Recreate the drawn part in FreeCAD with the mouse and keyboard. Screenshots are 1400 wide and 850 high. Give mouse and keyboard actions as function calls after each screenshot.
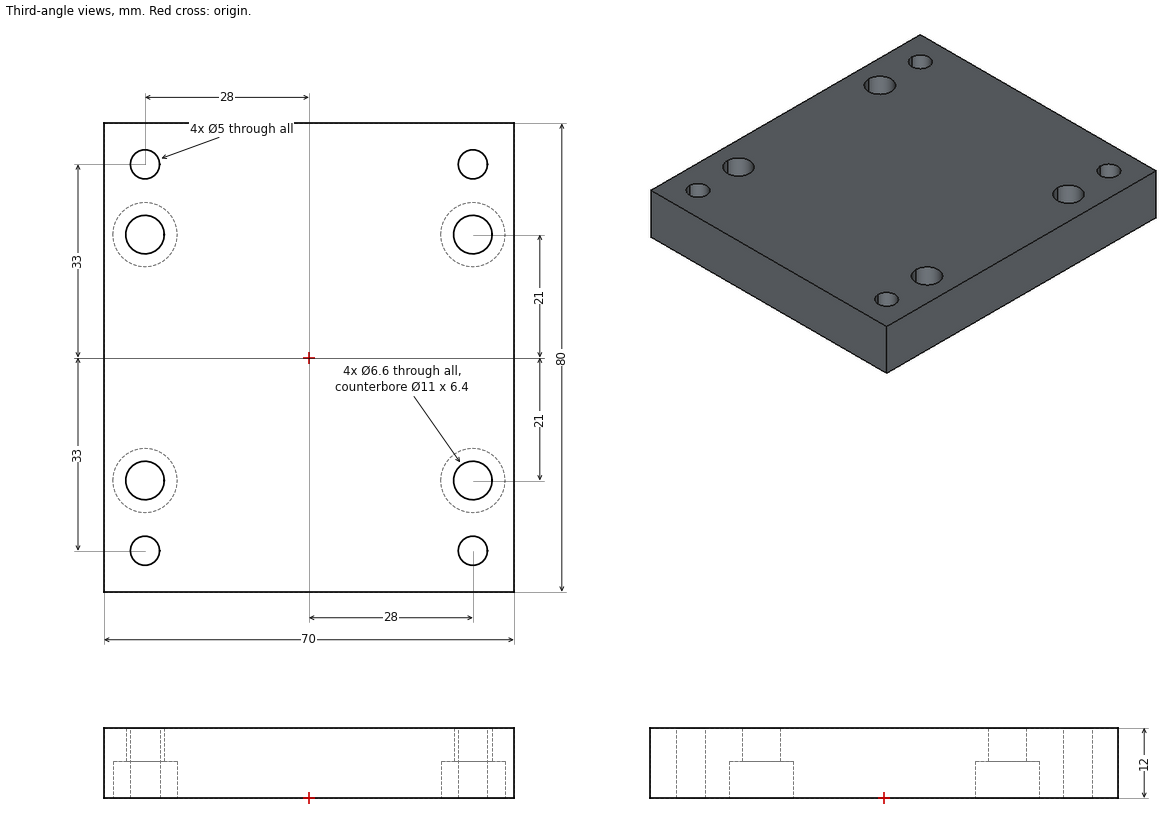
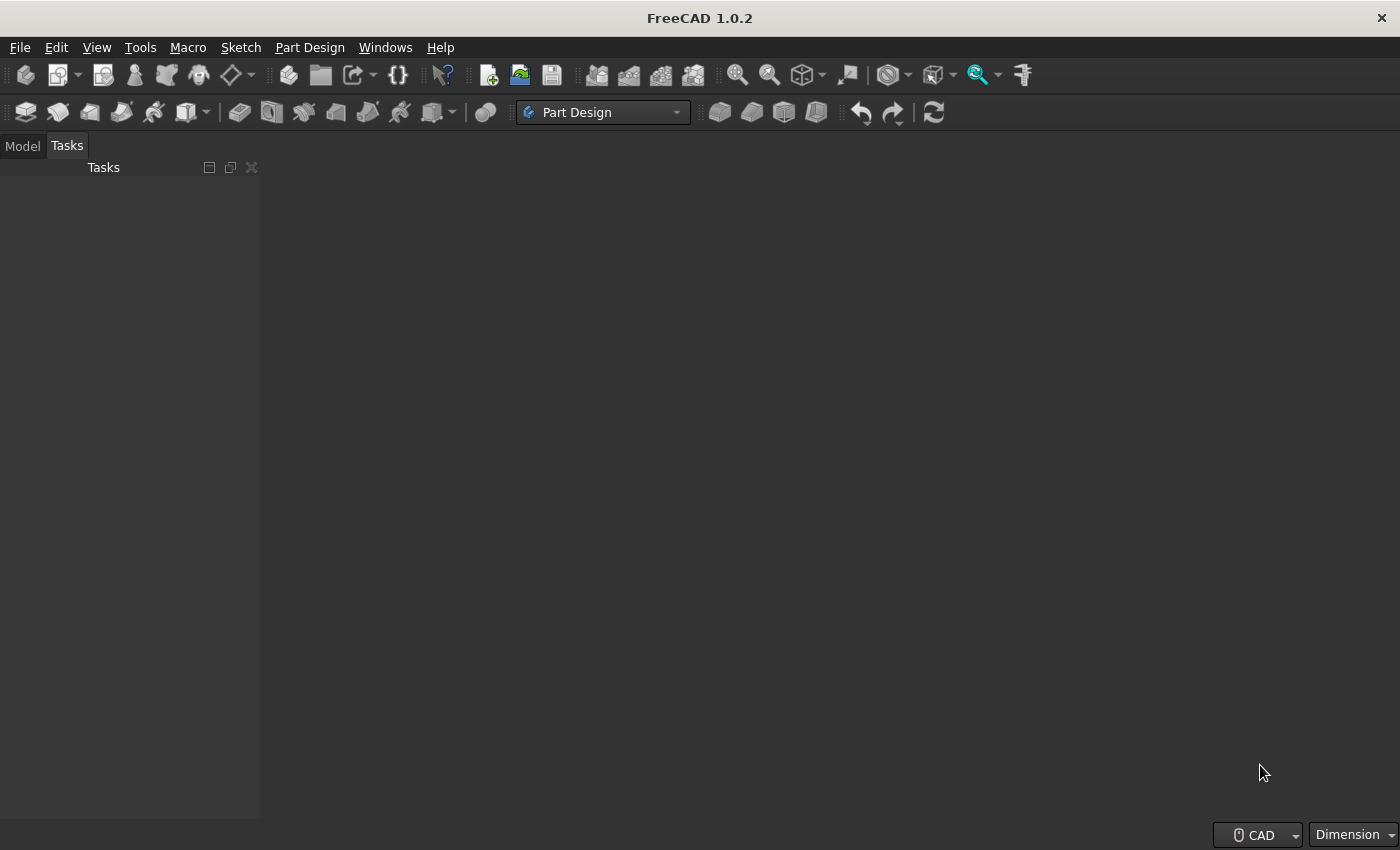
click(488, 76)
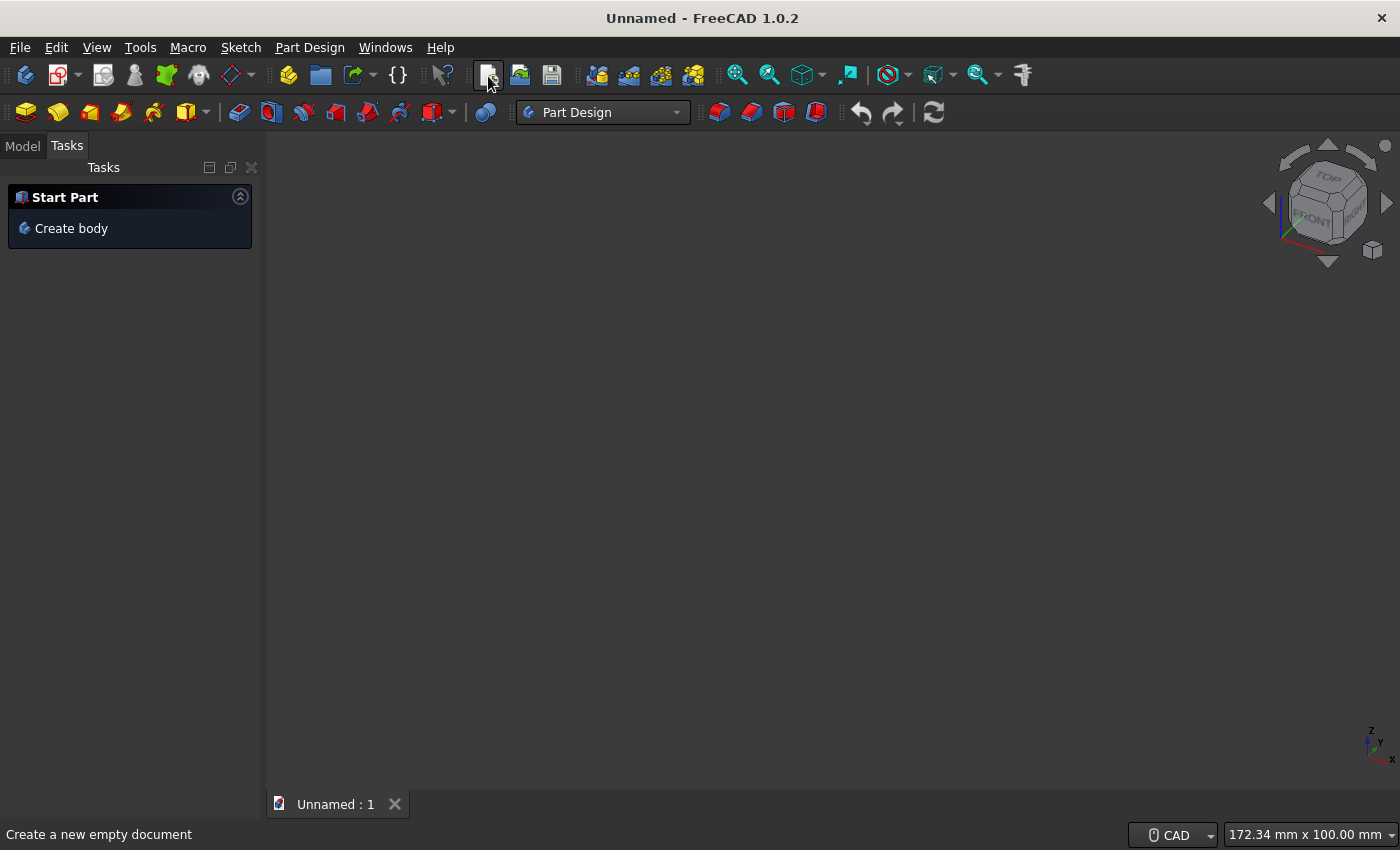
click(58, 76)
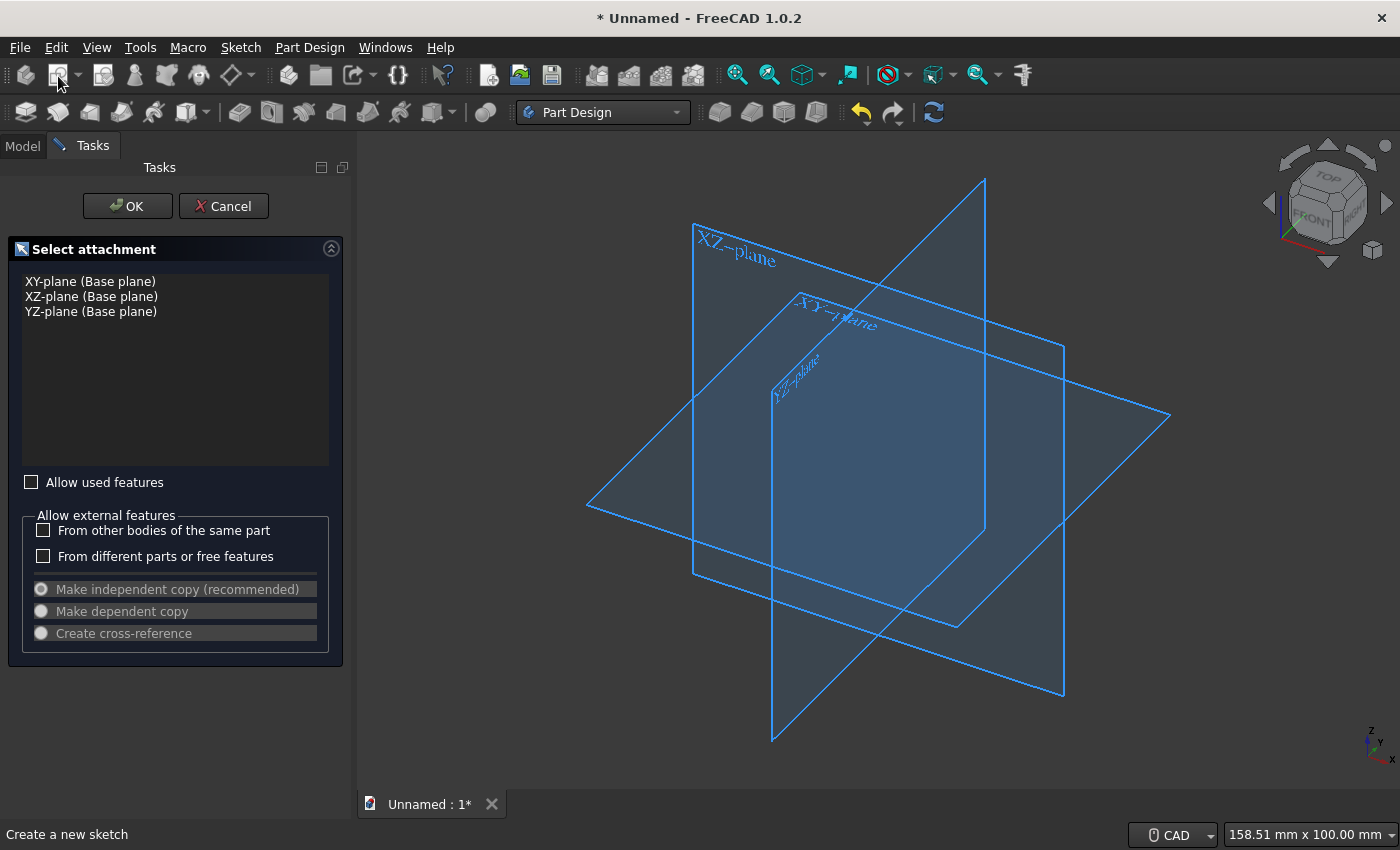
click(82, 282)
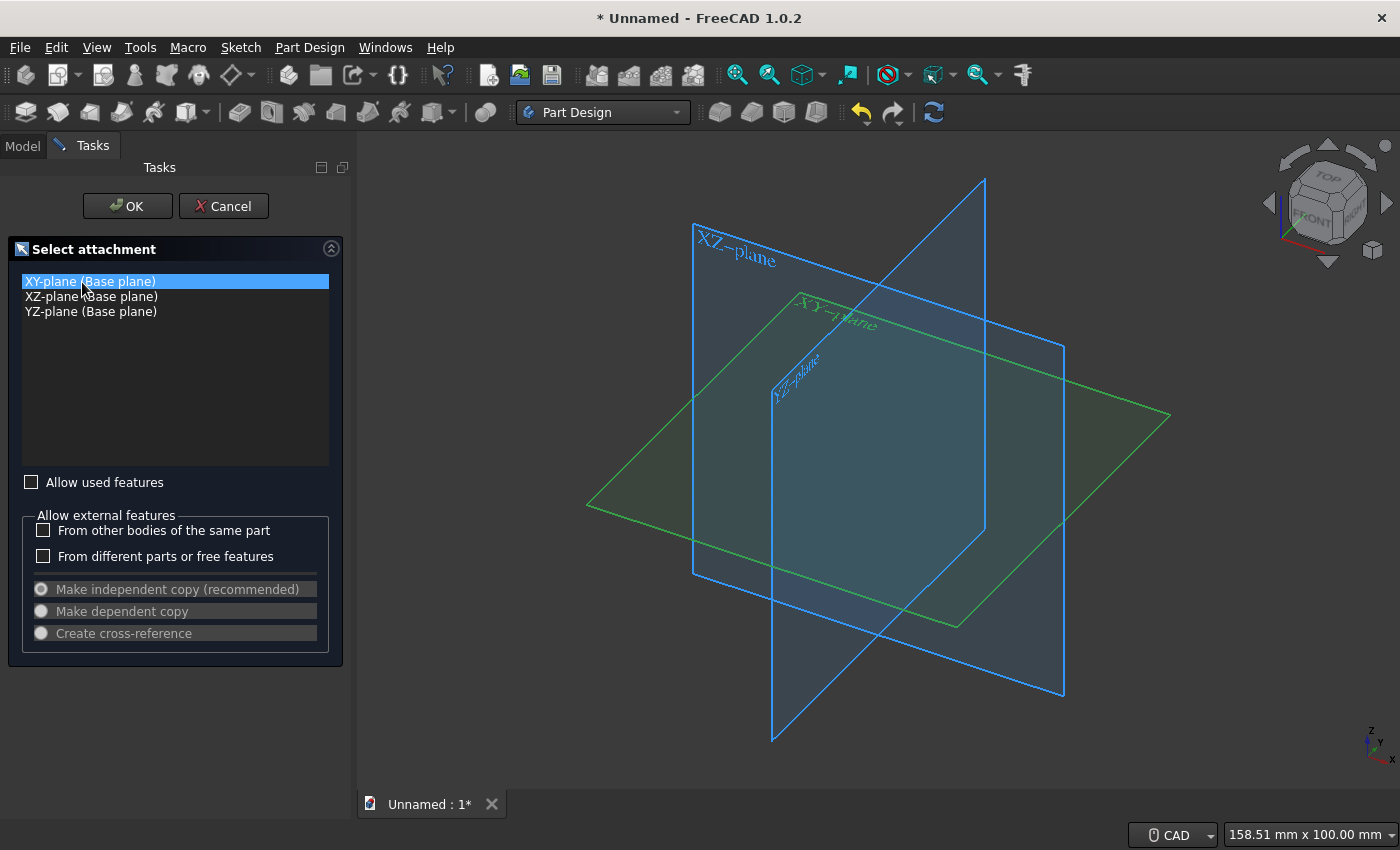
click(128, 206)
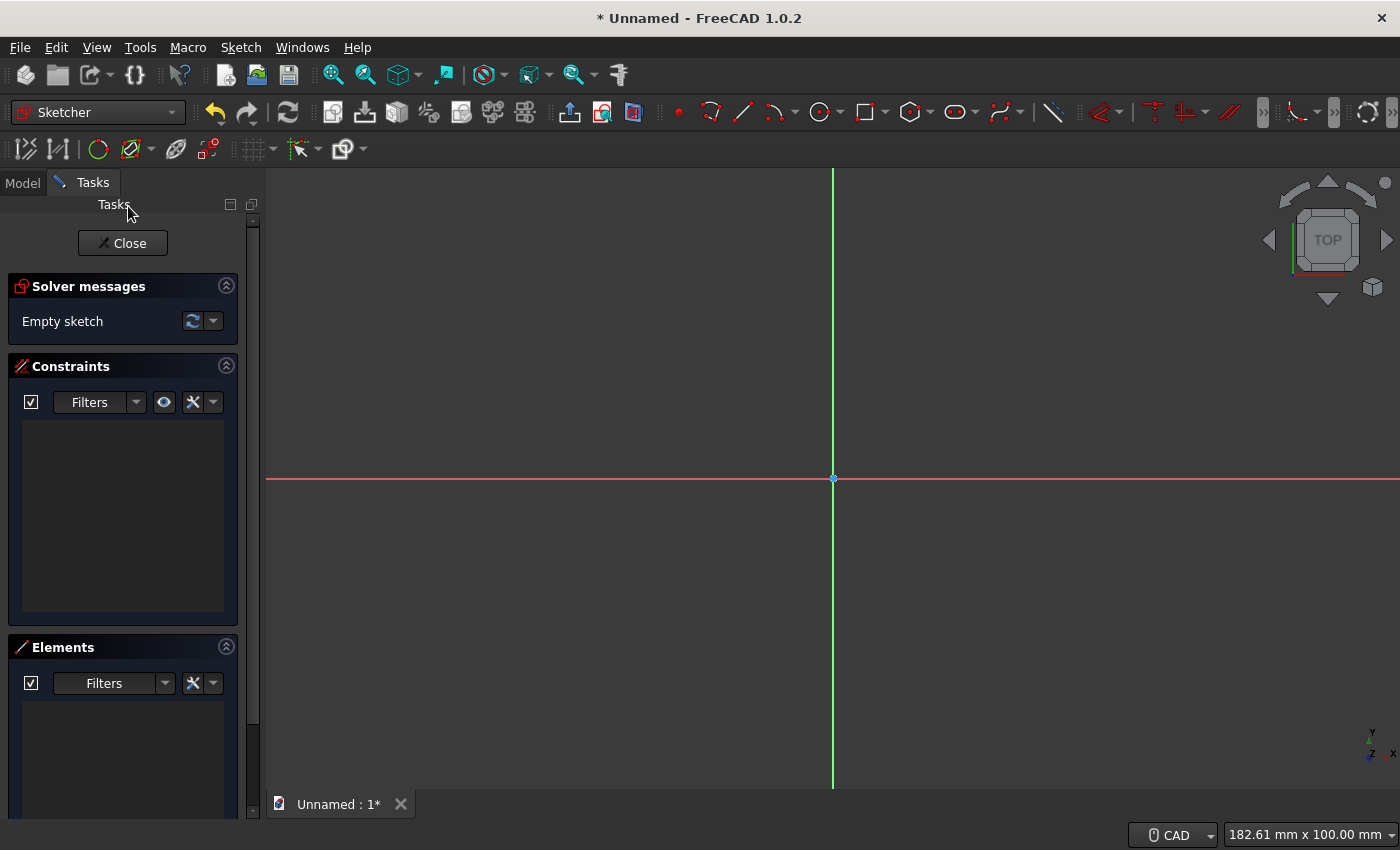
click(888, 112)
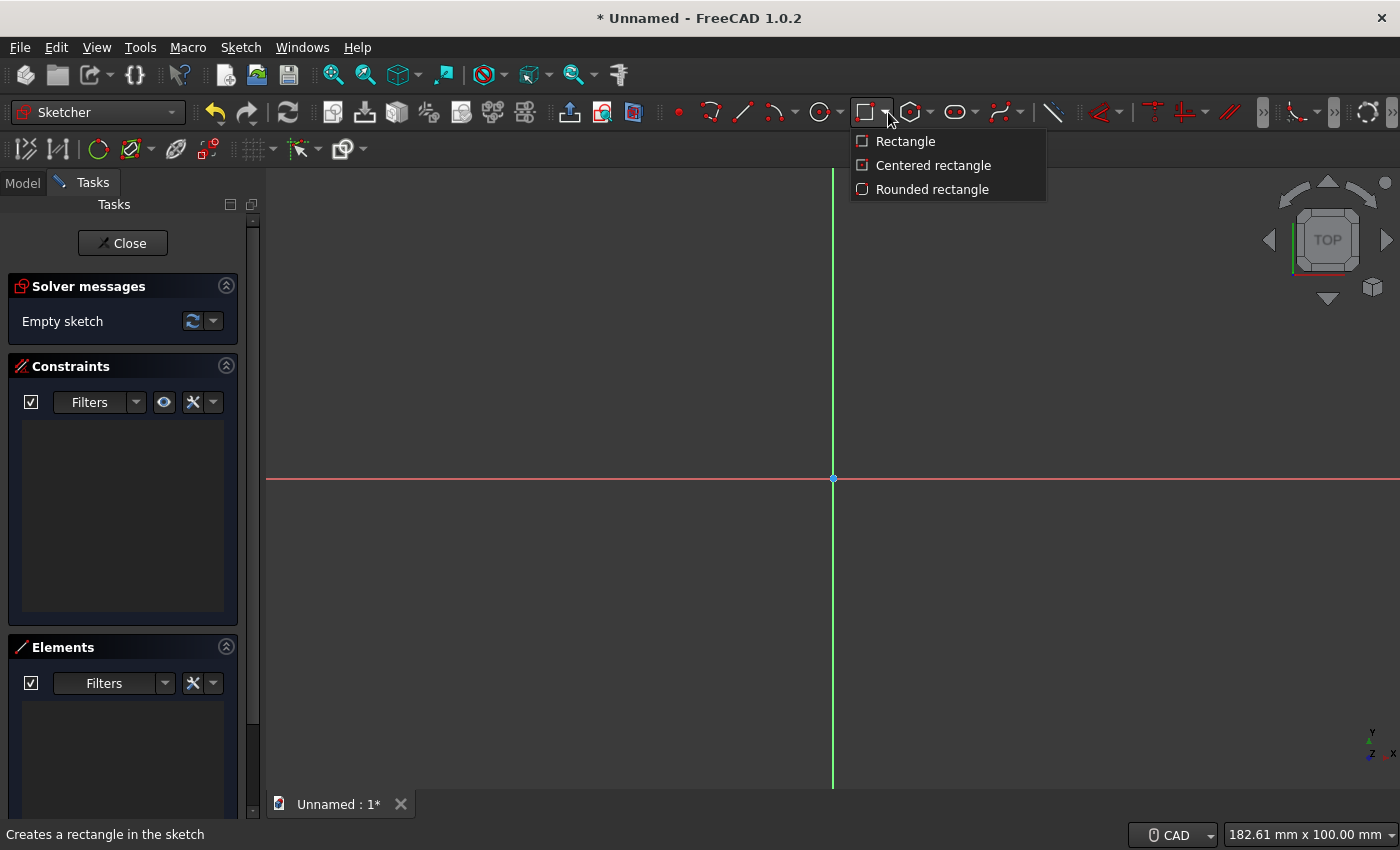
click(948, 165)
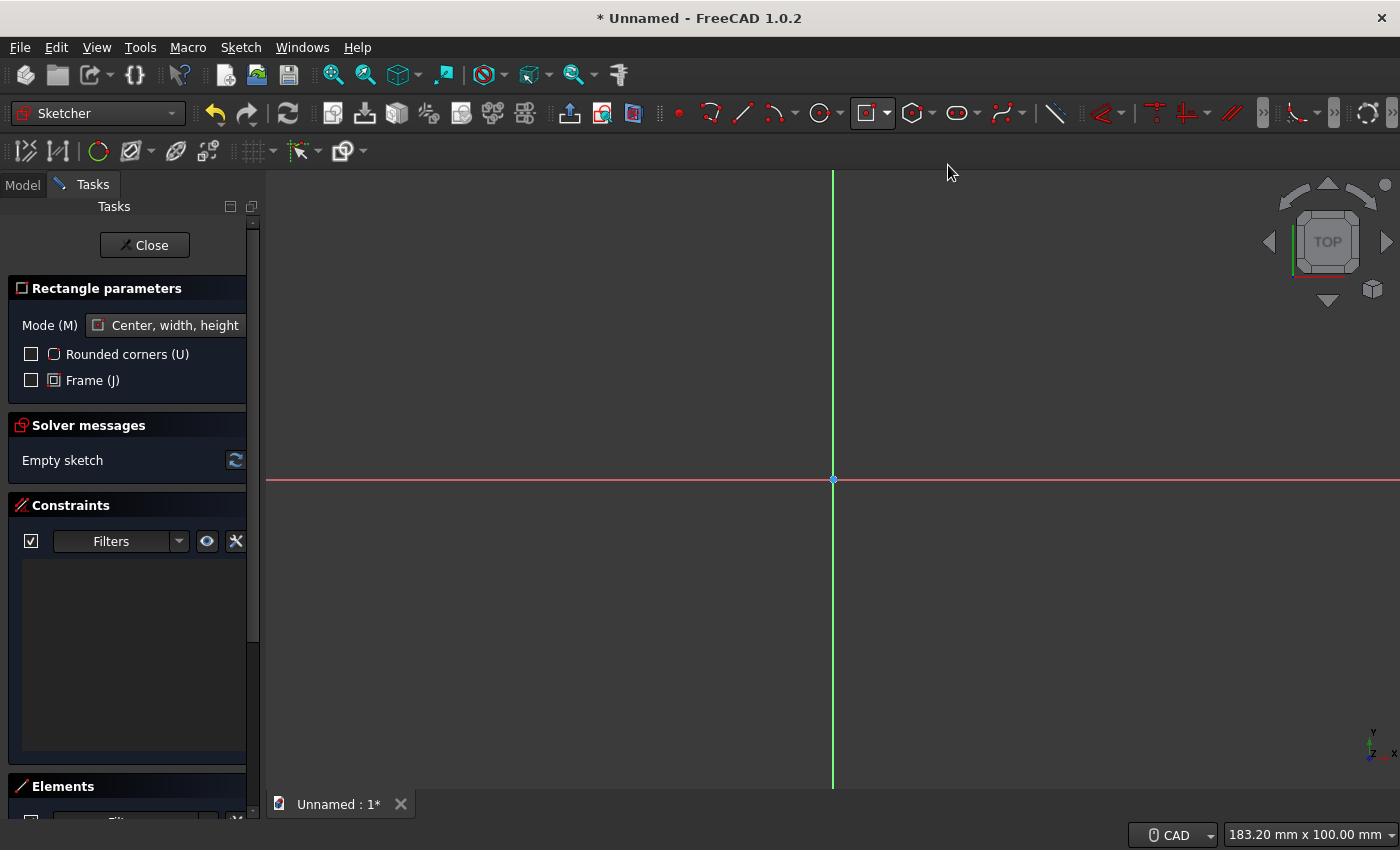
click(833, 480)
move(1050, 232)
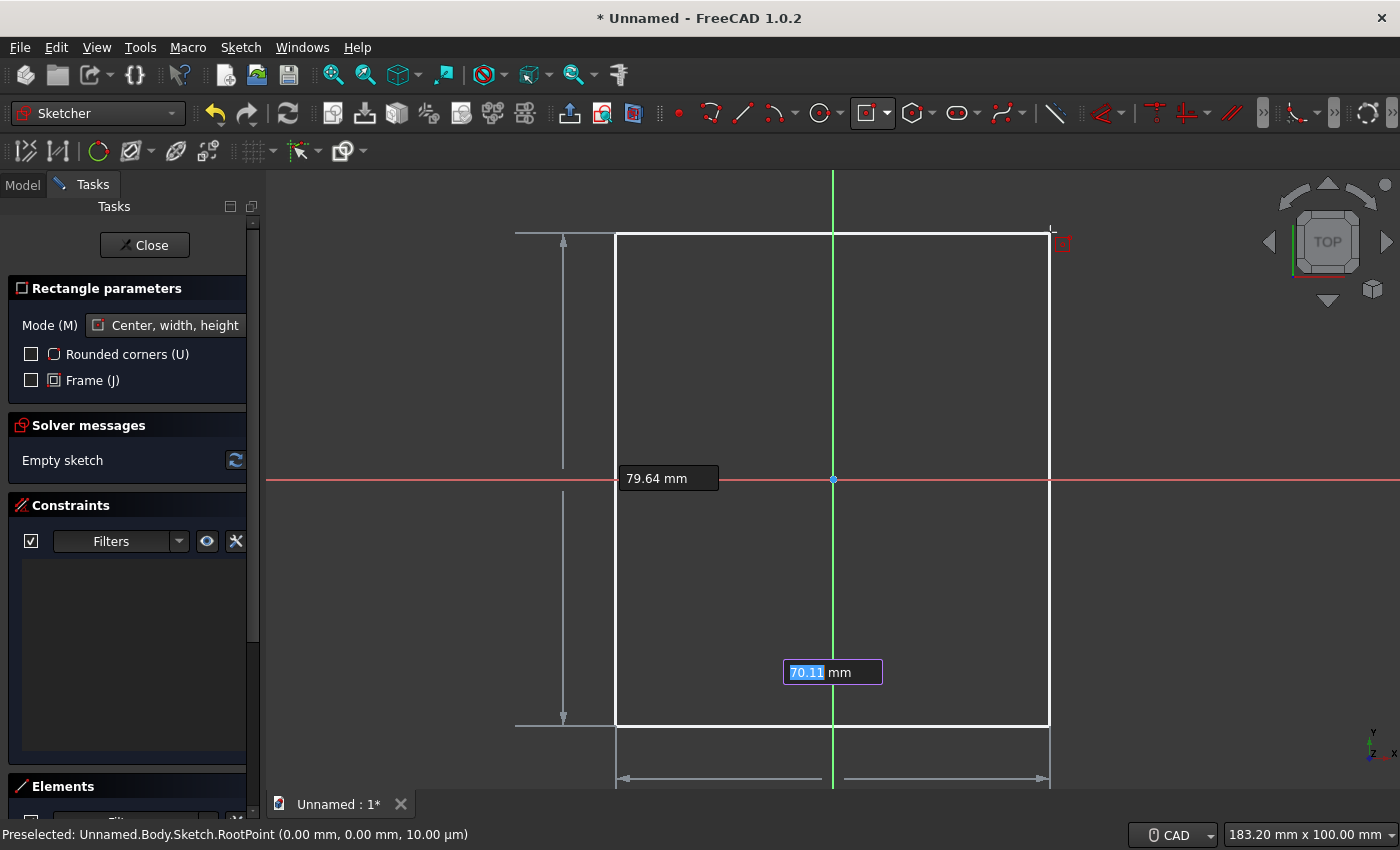
text(70)
key(Tab)
text(80)
key(Return)
key(Escape)